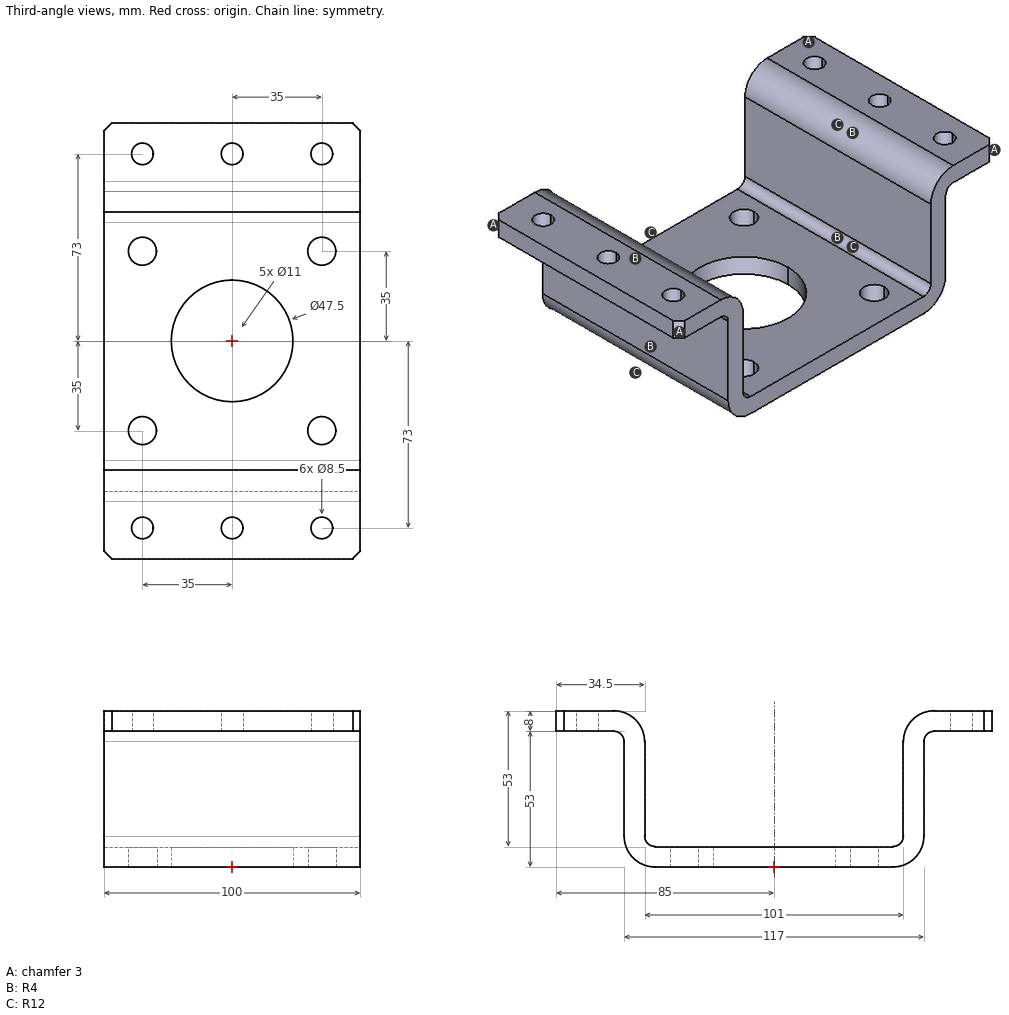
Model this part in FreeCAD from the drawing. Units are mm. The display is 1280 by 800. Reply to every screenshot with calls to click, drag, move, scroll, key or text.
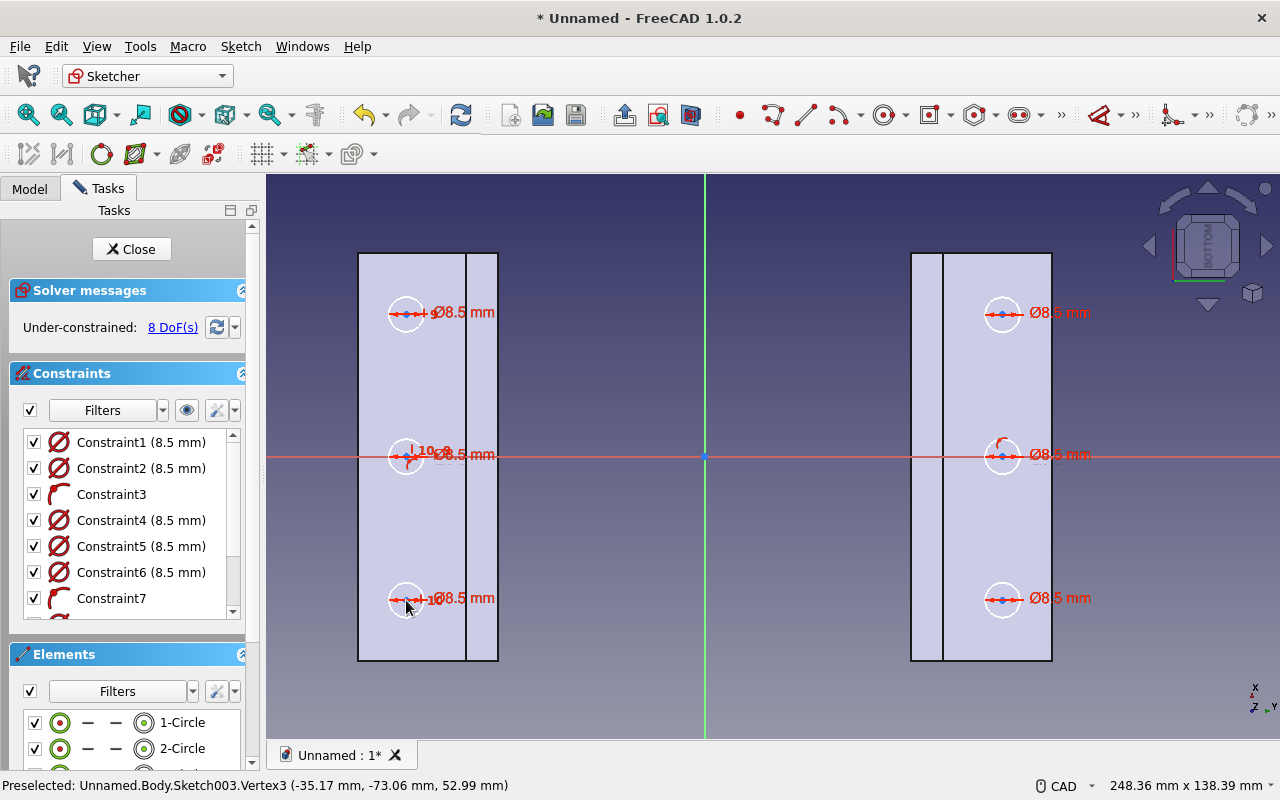
click(406, 600)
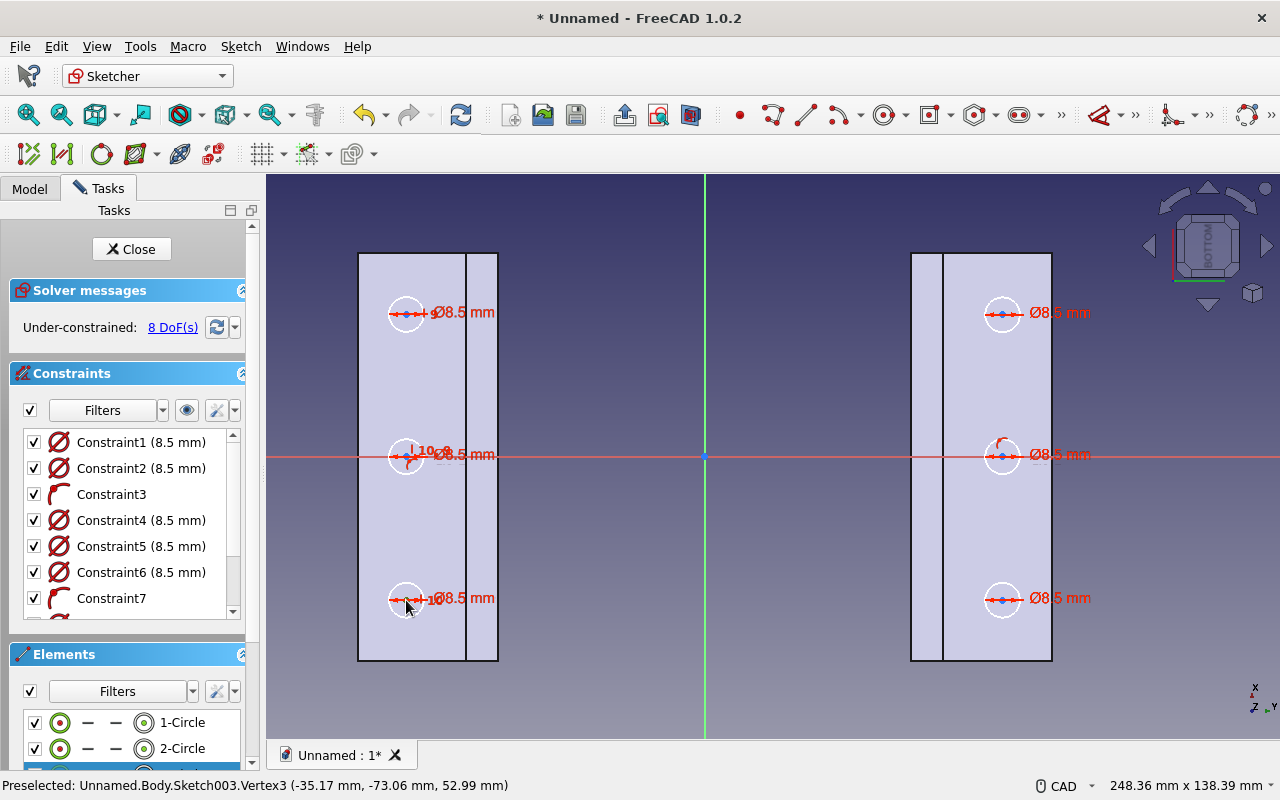
click(1003, 600)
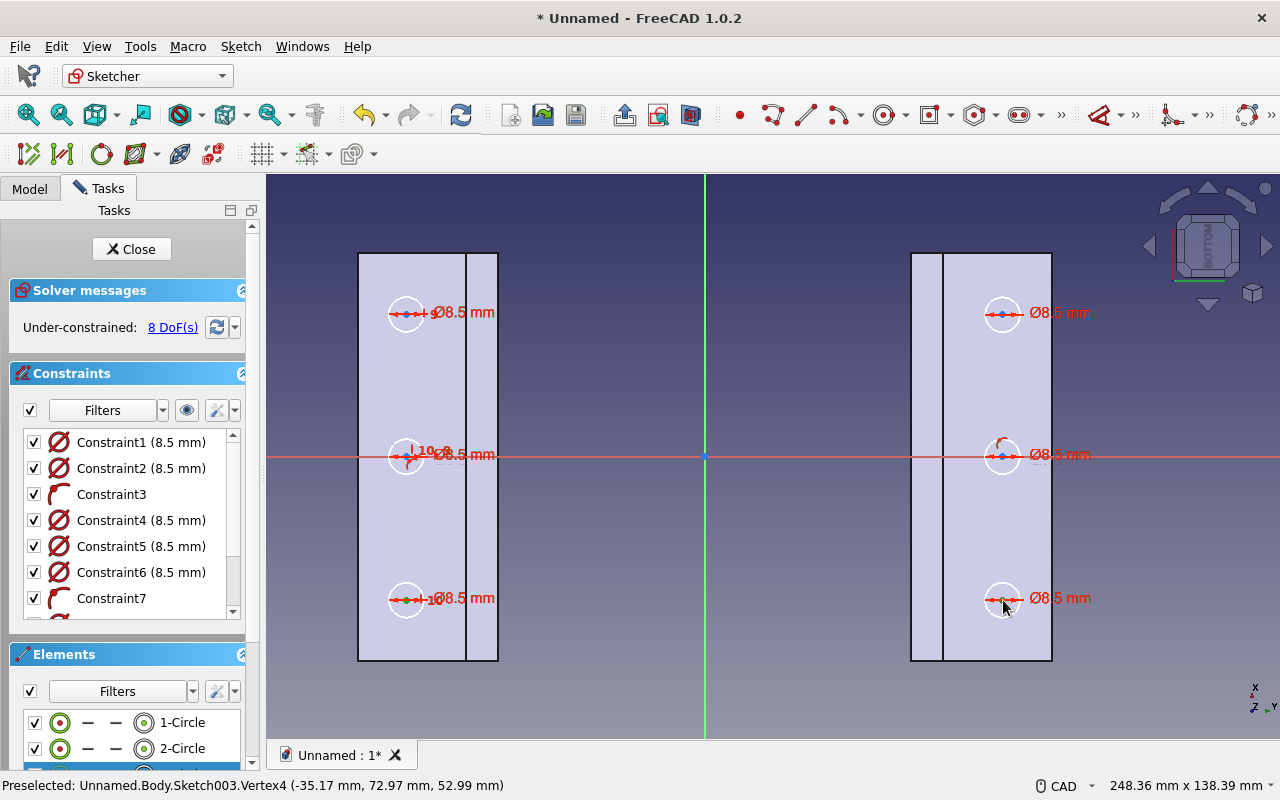
key(h)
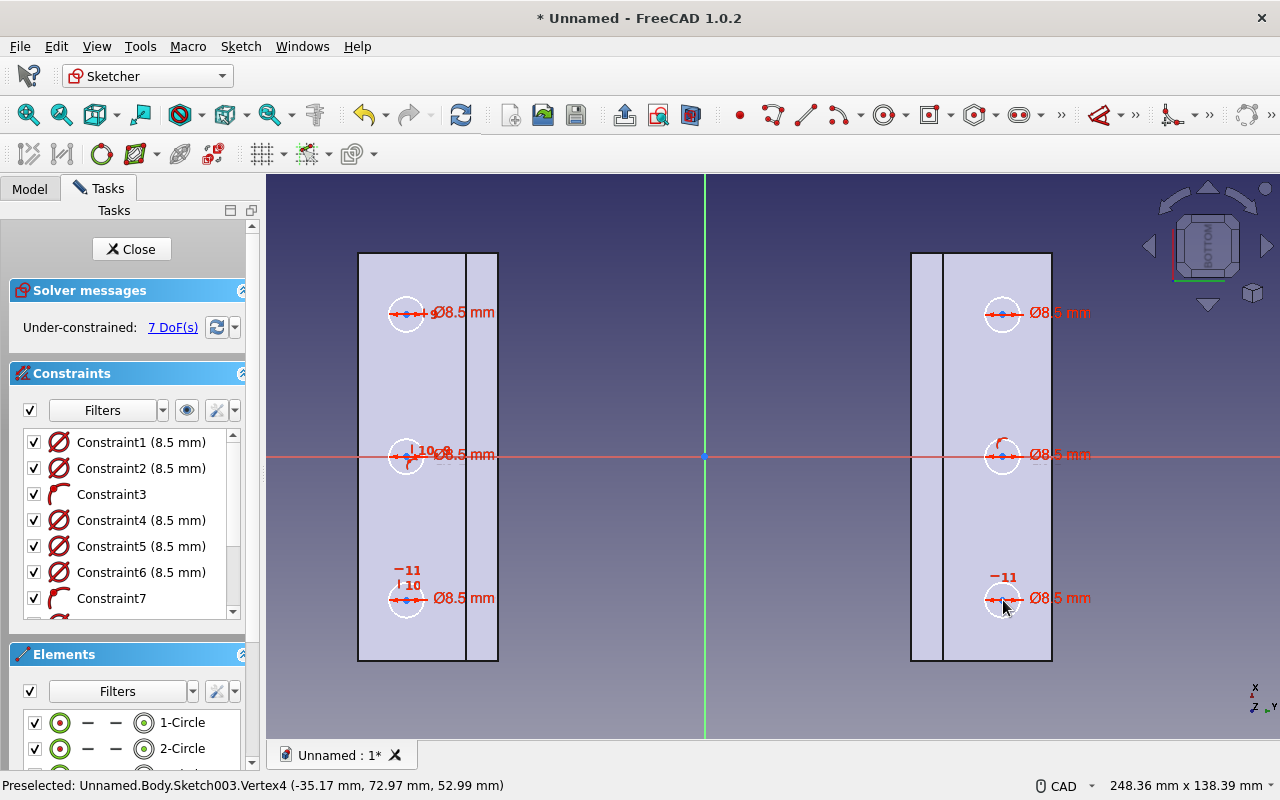
click(1003, 600)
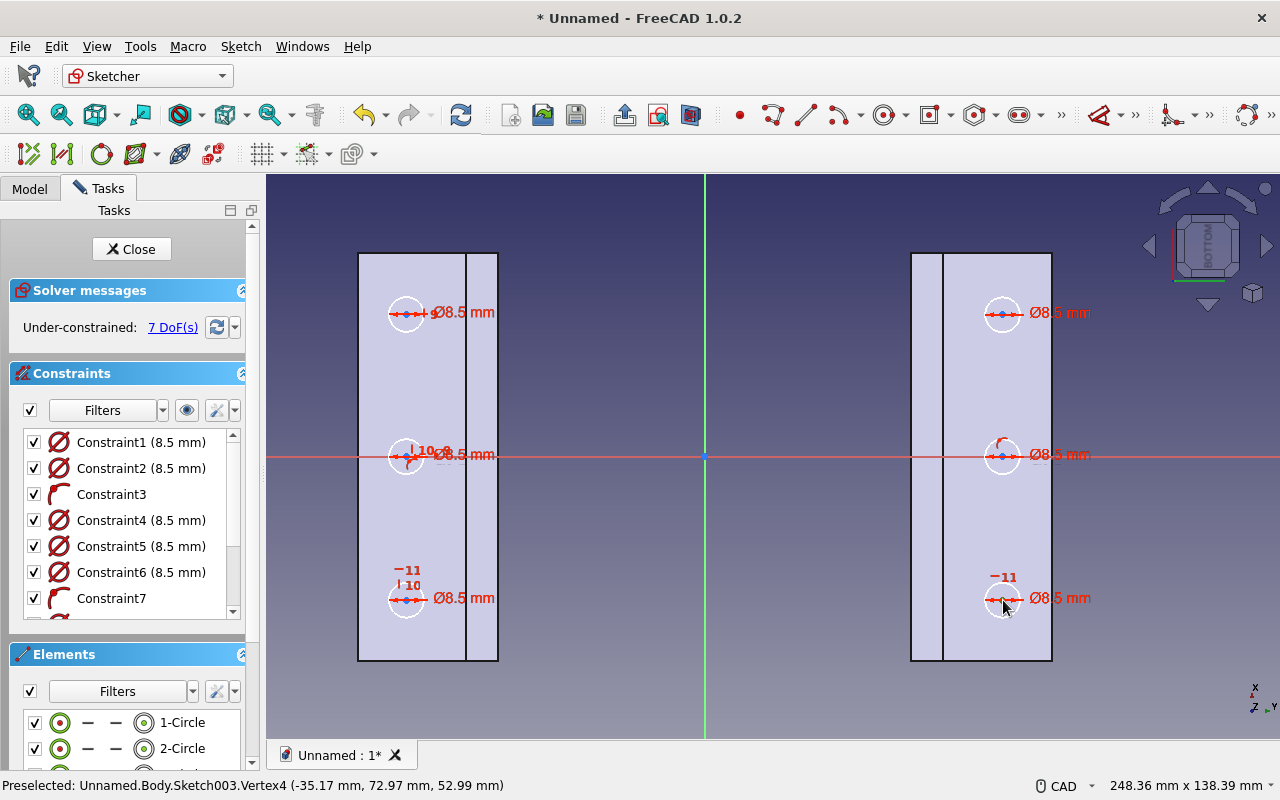
click(1003, 457)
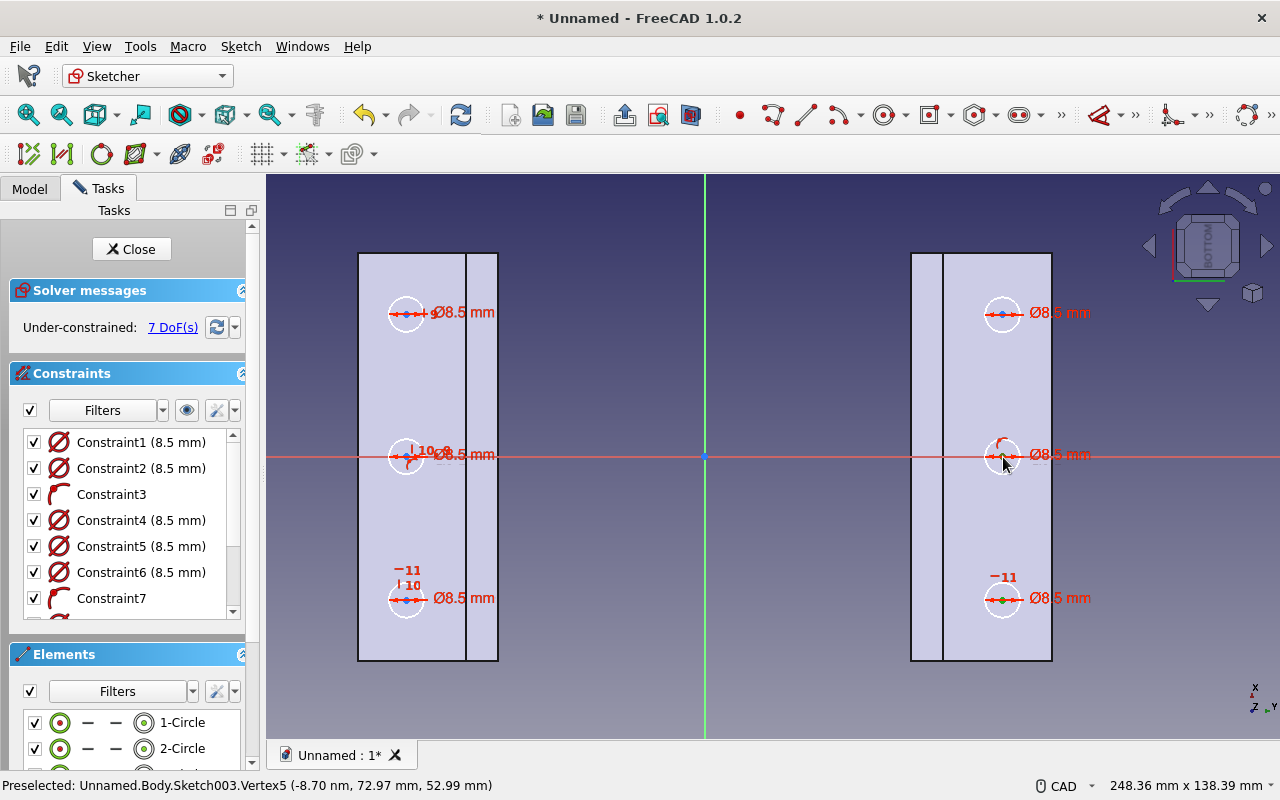
key(v)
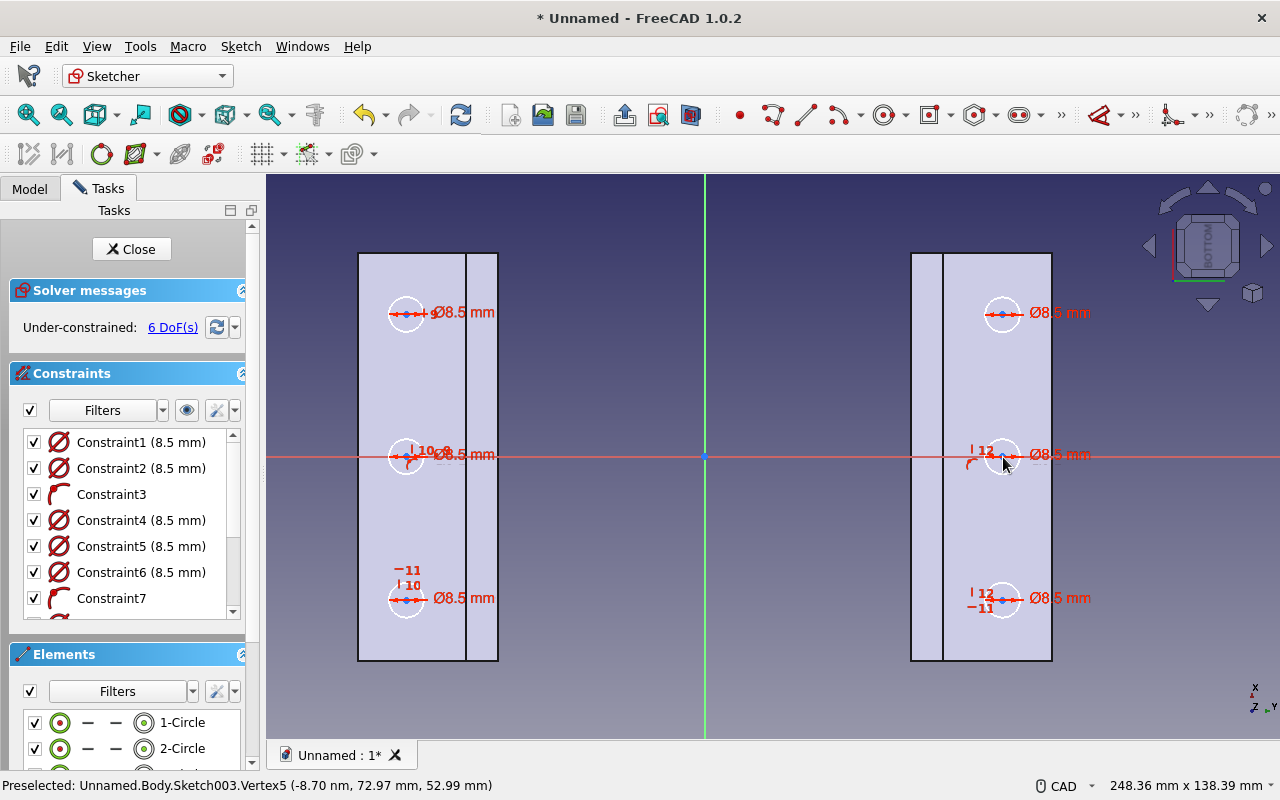
click(1003, 457)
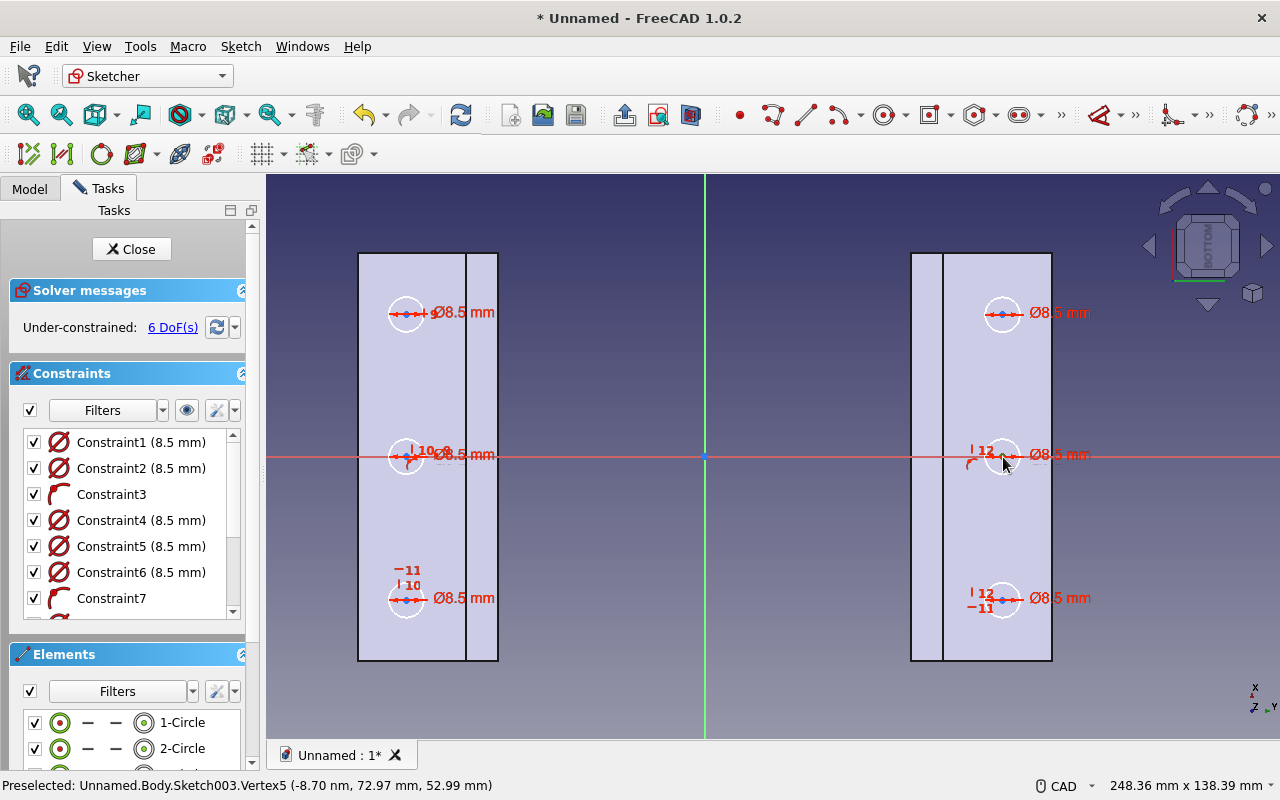
click(1003, 315)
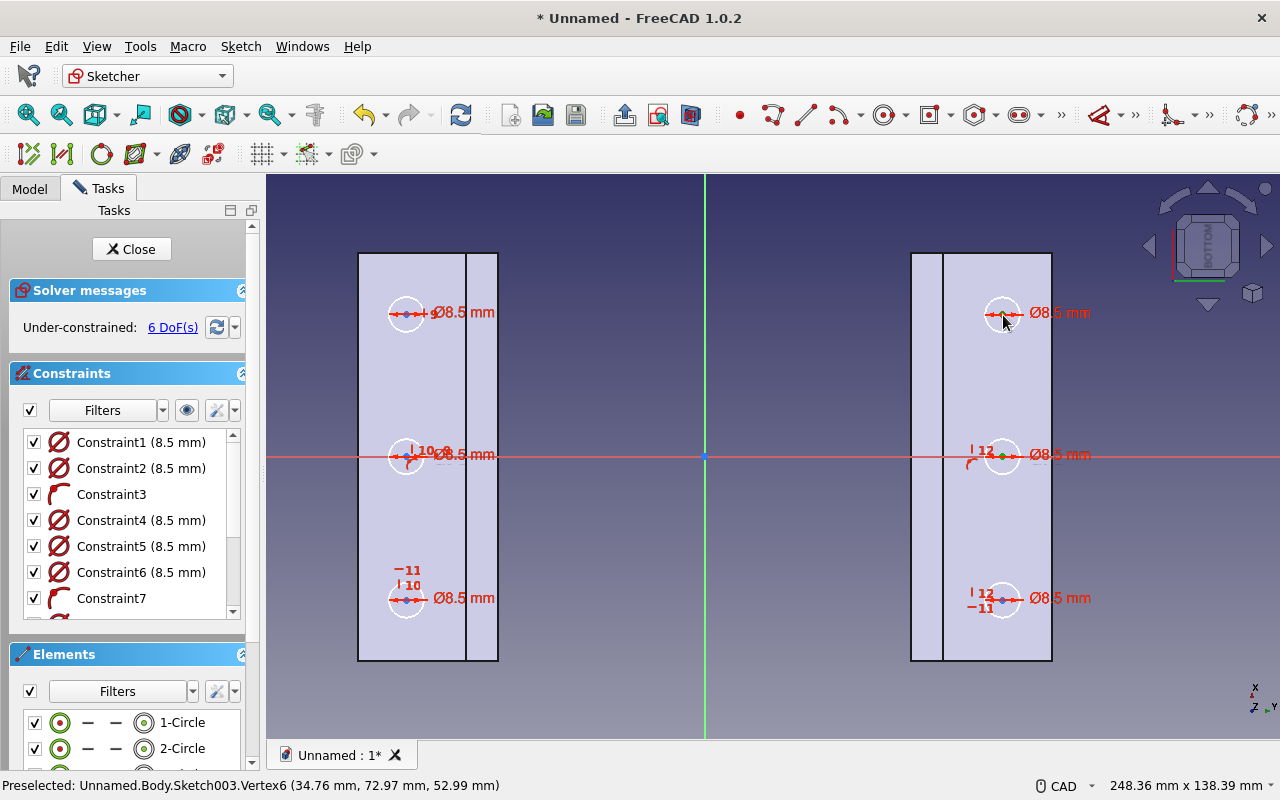
key(v)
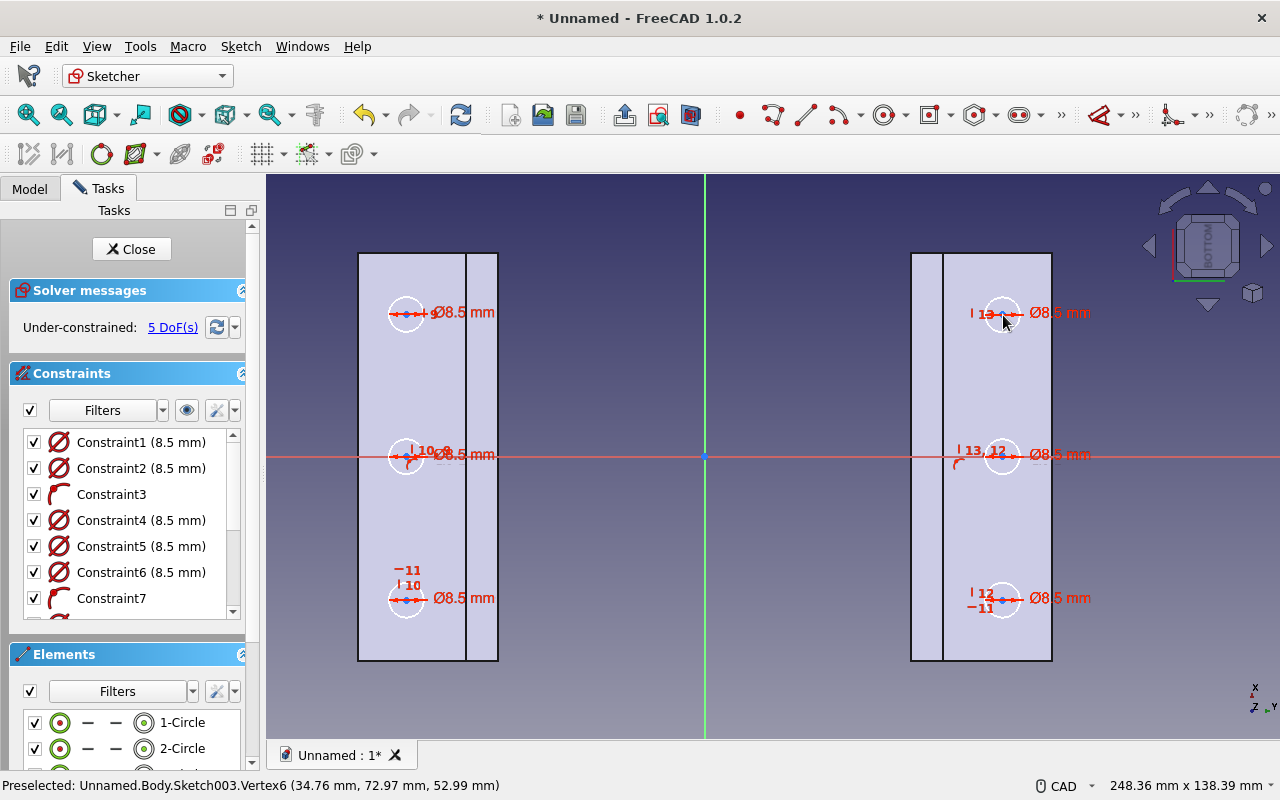
click(406, 314)